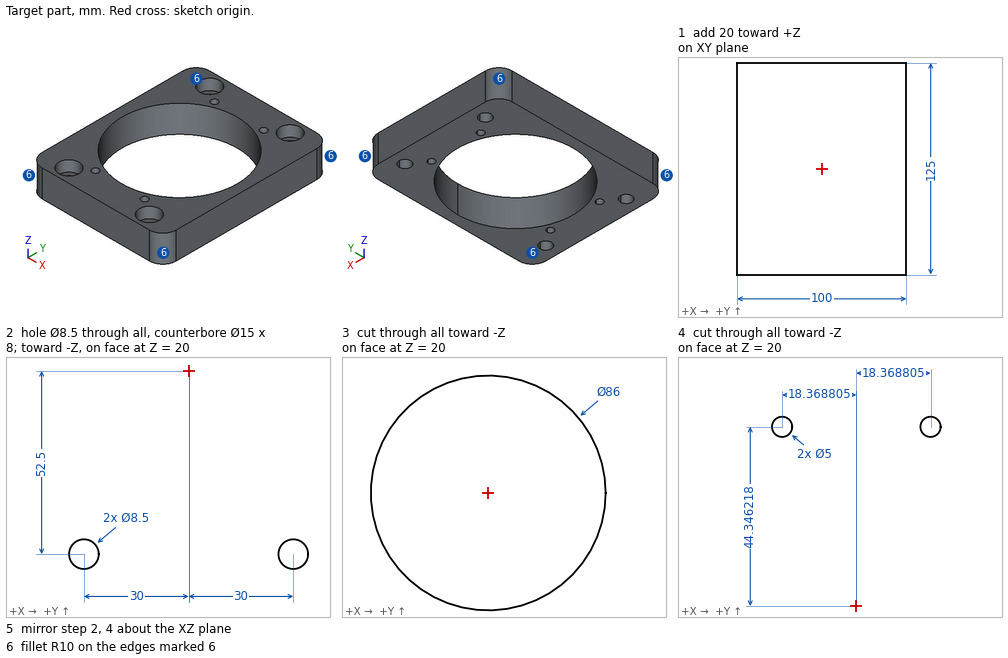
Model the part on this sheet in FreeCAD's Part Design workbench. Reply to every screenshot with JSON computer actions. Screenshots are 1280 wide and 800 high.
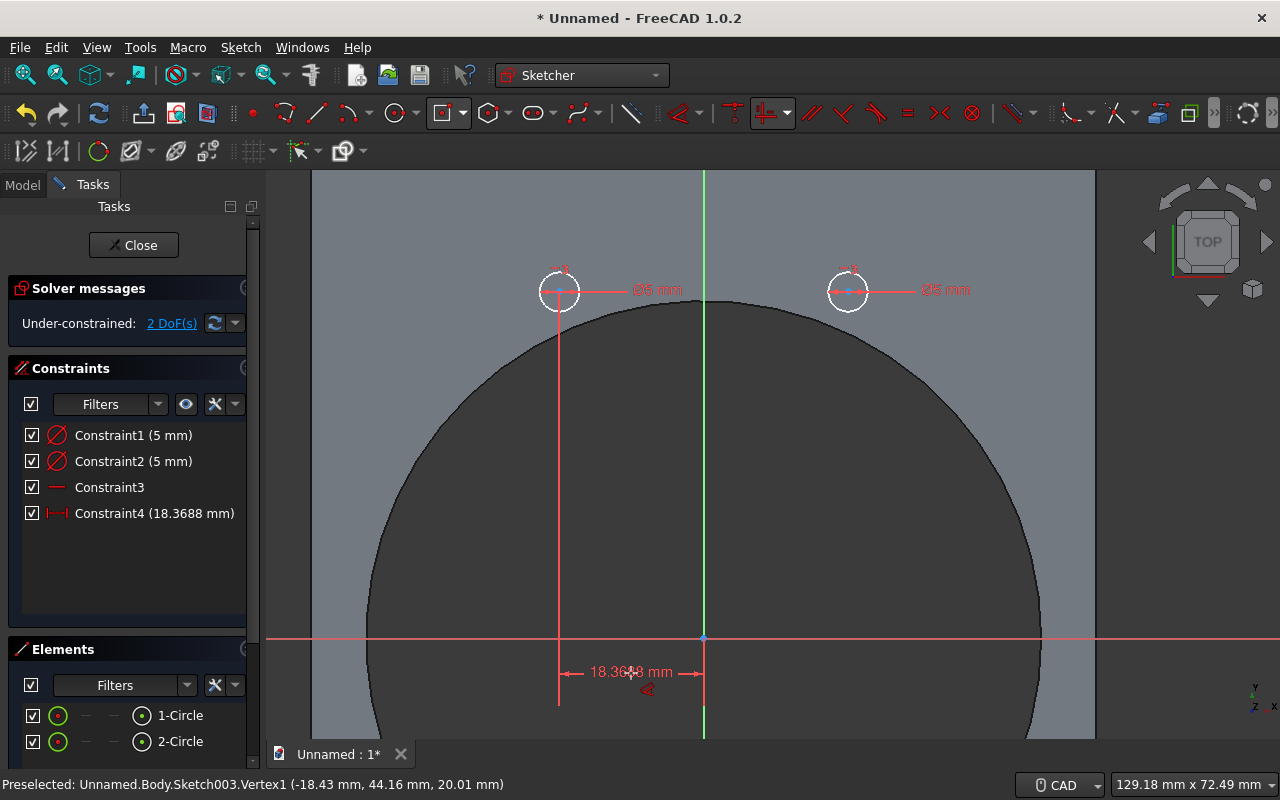
{"action": "left_click", "coordinate": [559, 292]}
{"action": "left_click", "coordinate": [525, 465]}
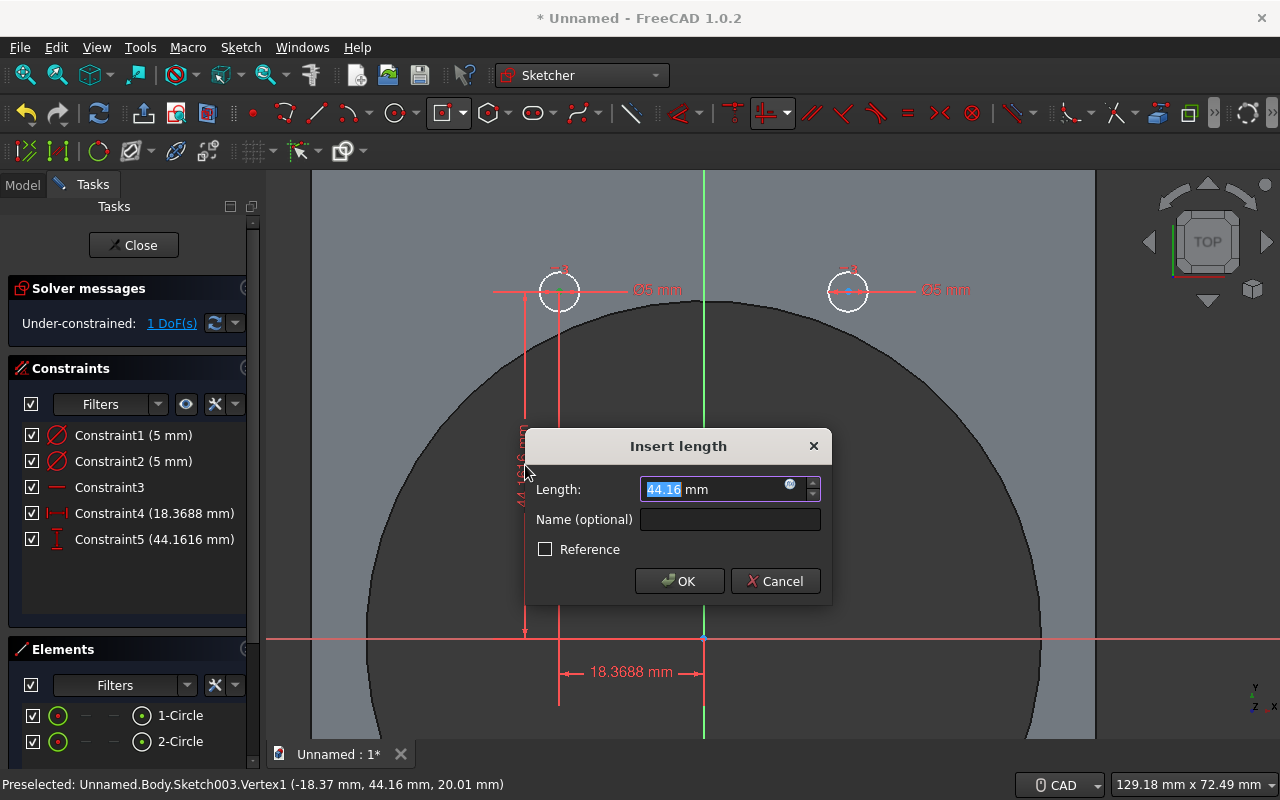
{"action": "type", "text": "44.346218"}
{"action": "key", "text": "Return"}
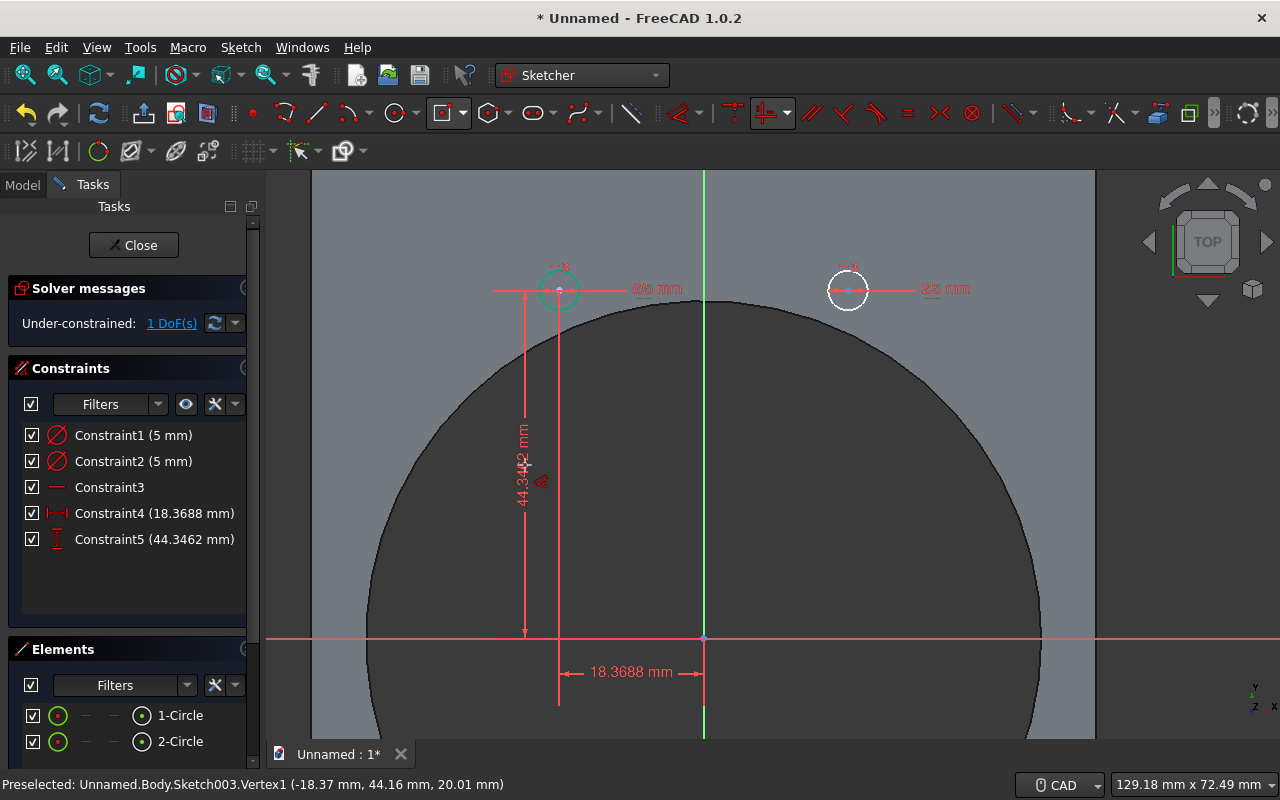
{"action": "left_click", "coordinate": [848, 291]}
{"action": "left_click", "coordinate": [776, 673]}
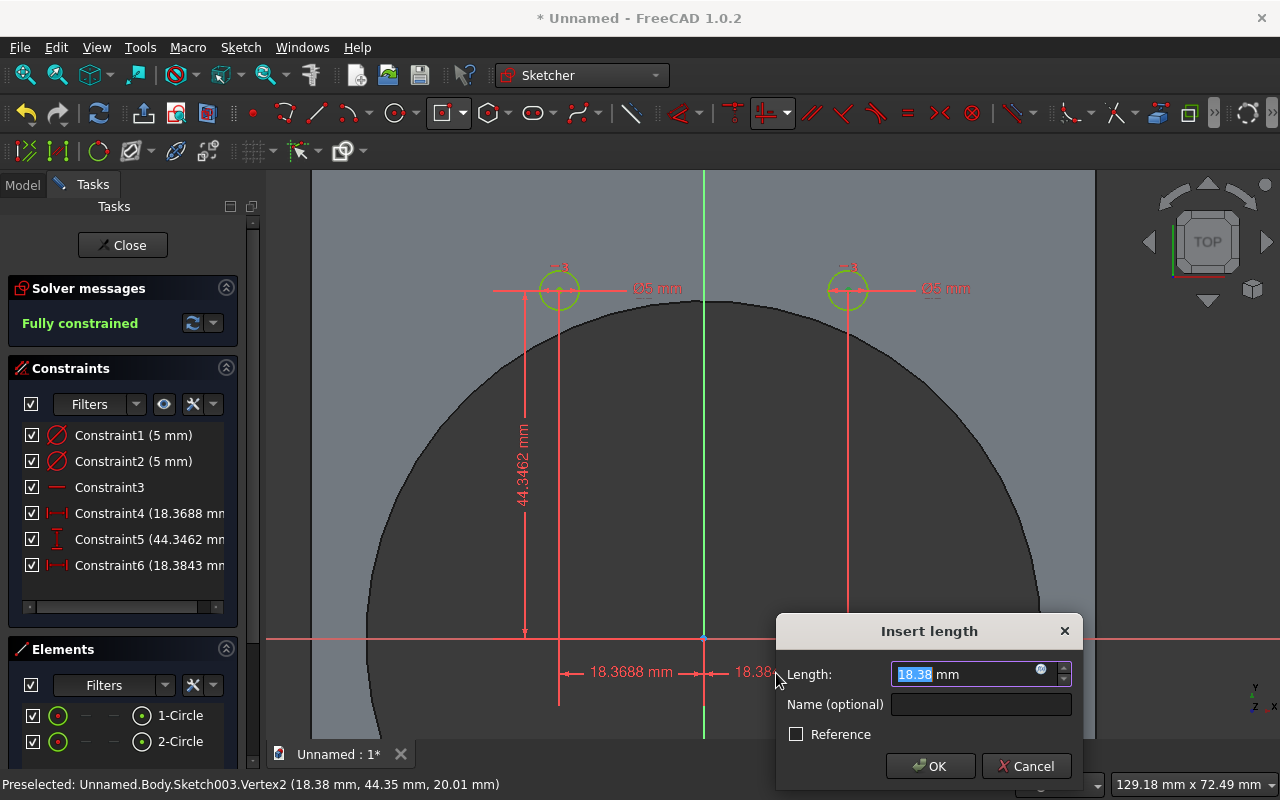
{"action": "type", "text": "18.368805"}
{"action": "key", "text": "Return"}
{"action": "key", "text": "Escape"}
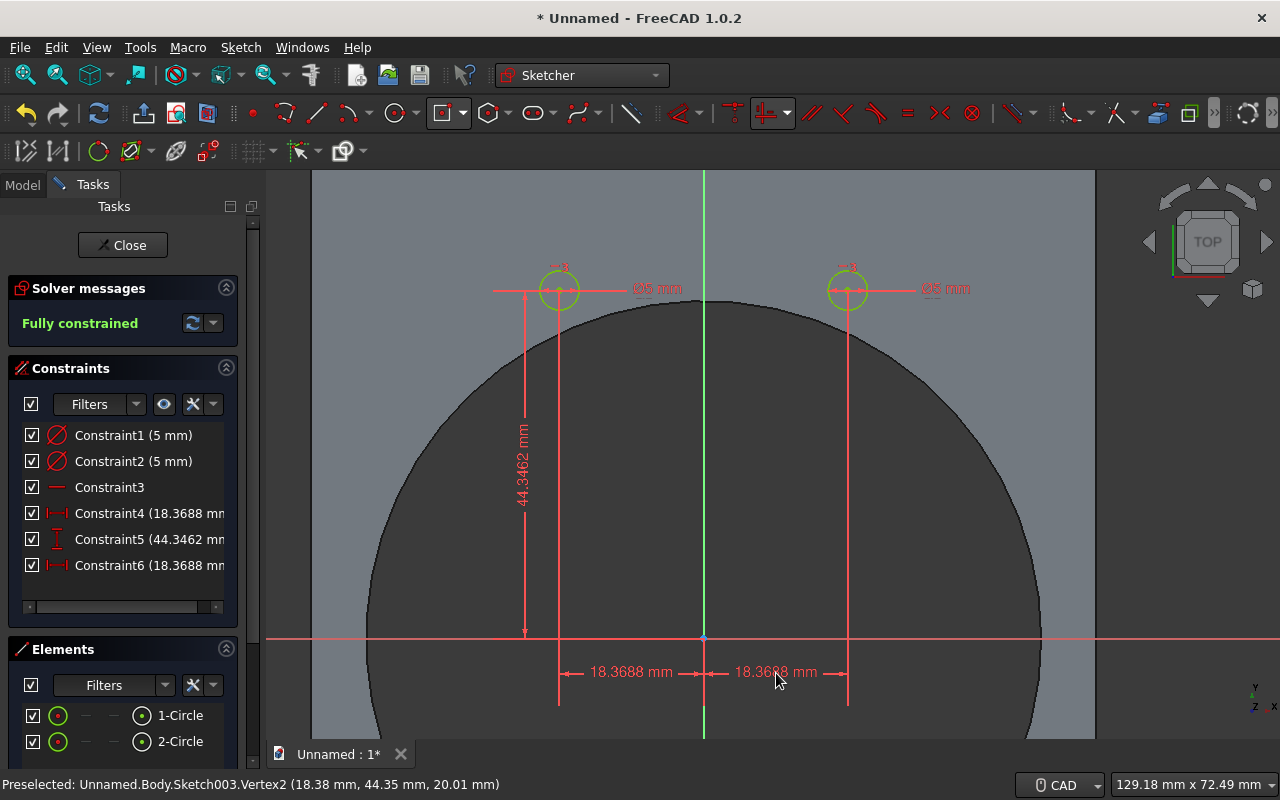
{"action": "left_click", "coordinate": [123, 245]}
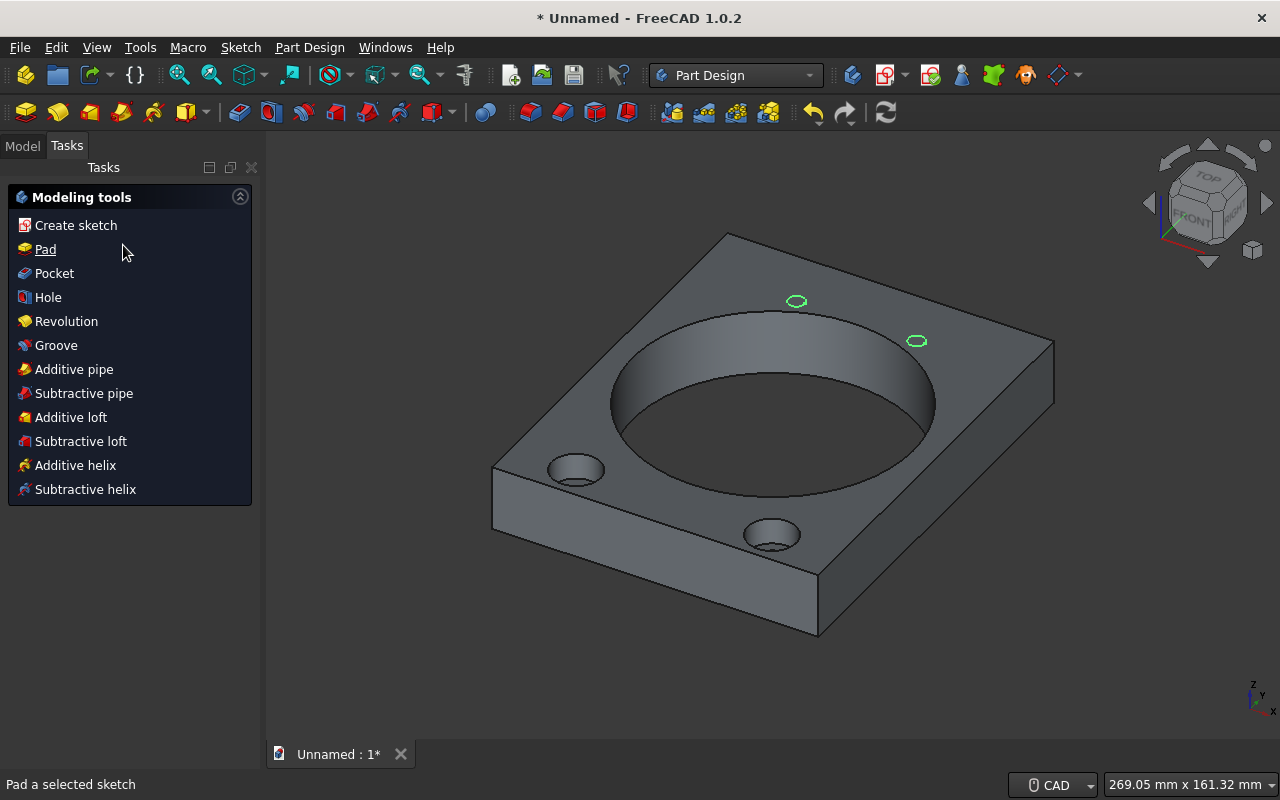
{"action": "left_click", "coordinate": [240, 112]}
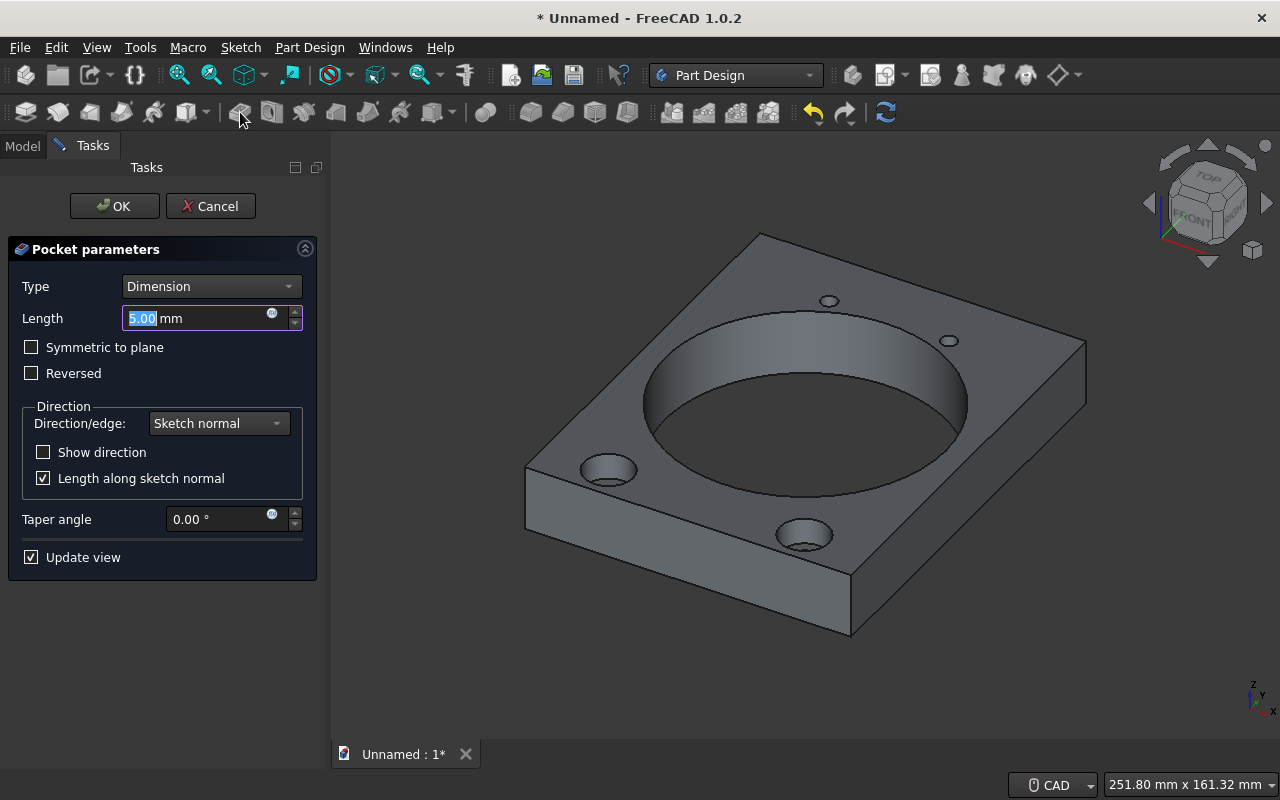
{"action": "left_click", "coordinate": [212, 286]}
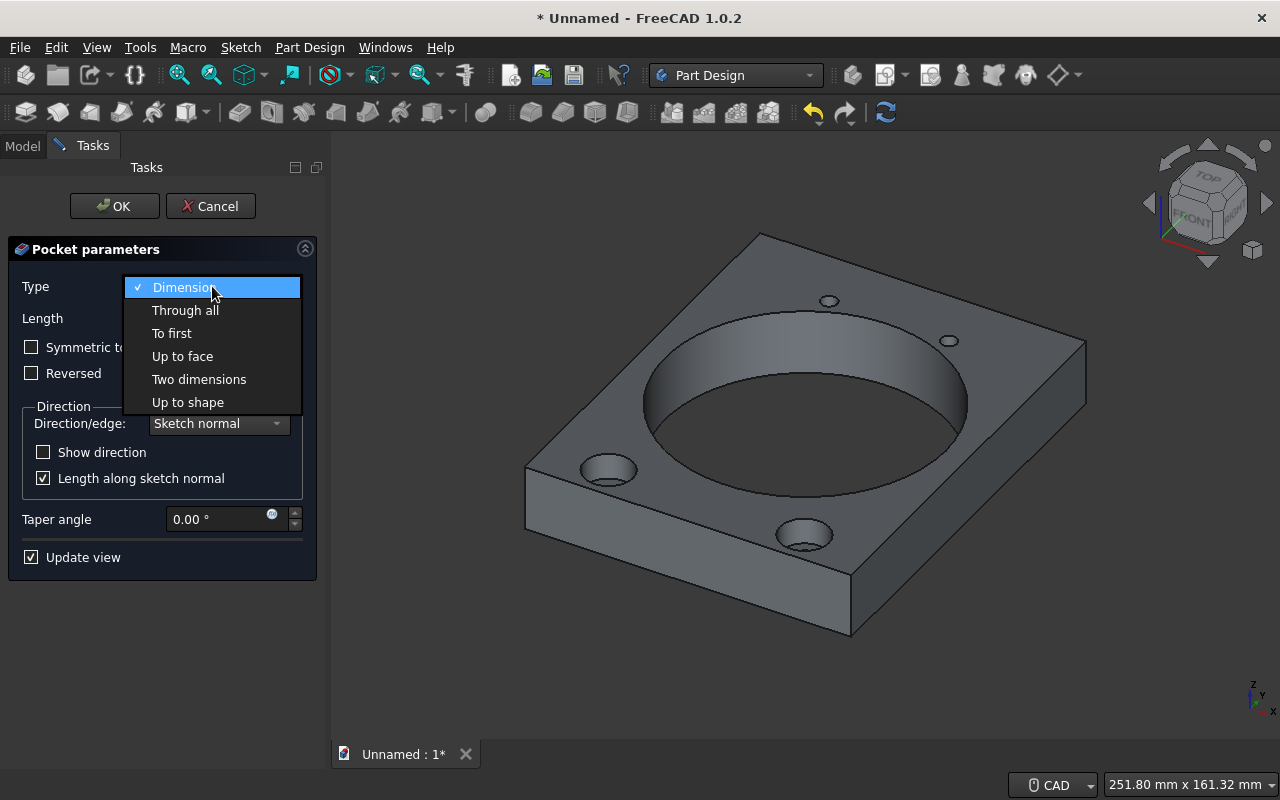
{"action": "left_click", "coordinate": [212, 310]}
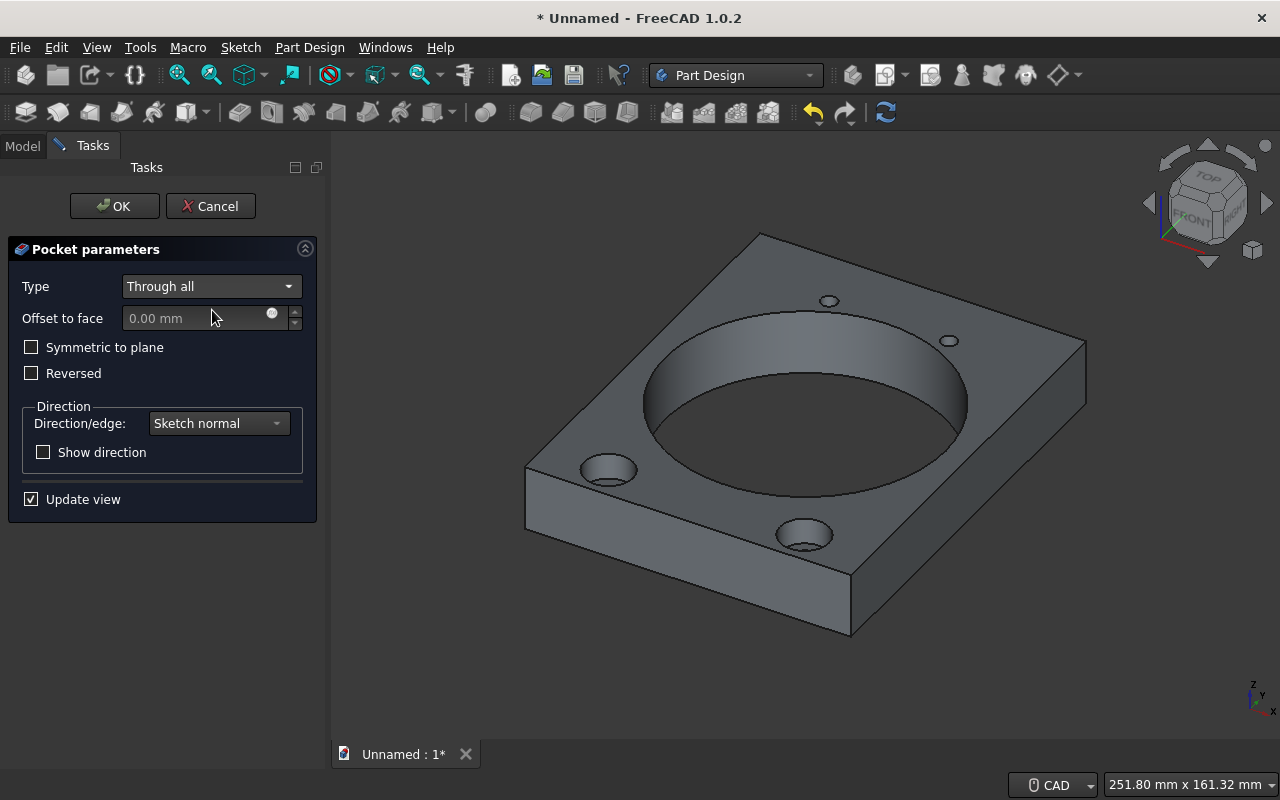
{"action": "left_click", "coordinate": [115, 206]}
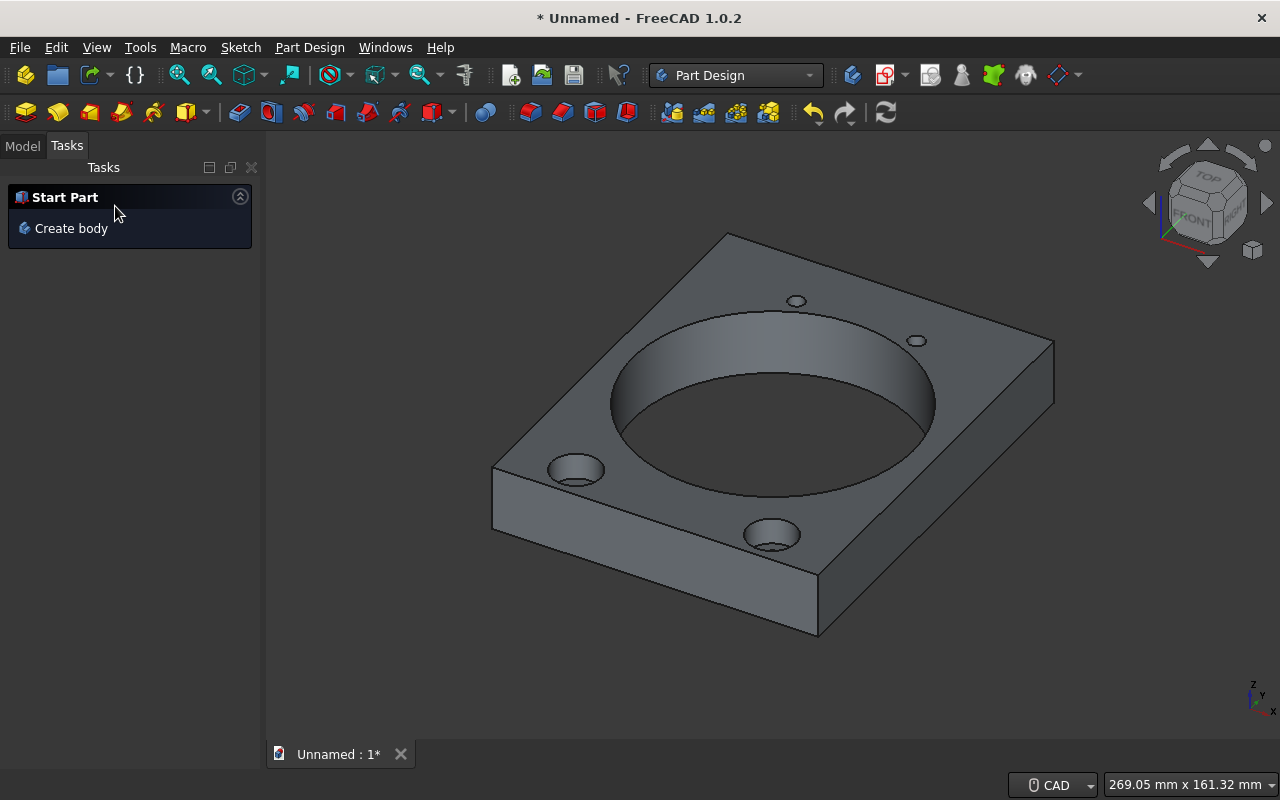
{"action": "left_click", "coordinate": [23, 145]}